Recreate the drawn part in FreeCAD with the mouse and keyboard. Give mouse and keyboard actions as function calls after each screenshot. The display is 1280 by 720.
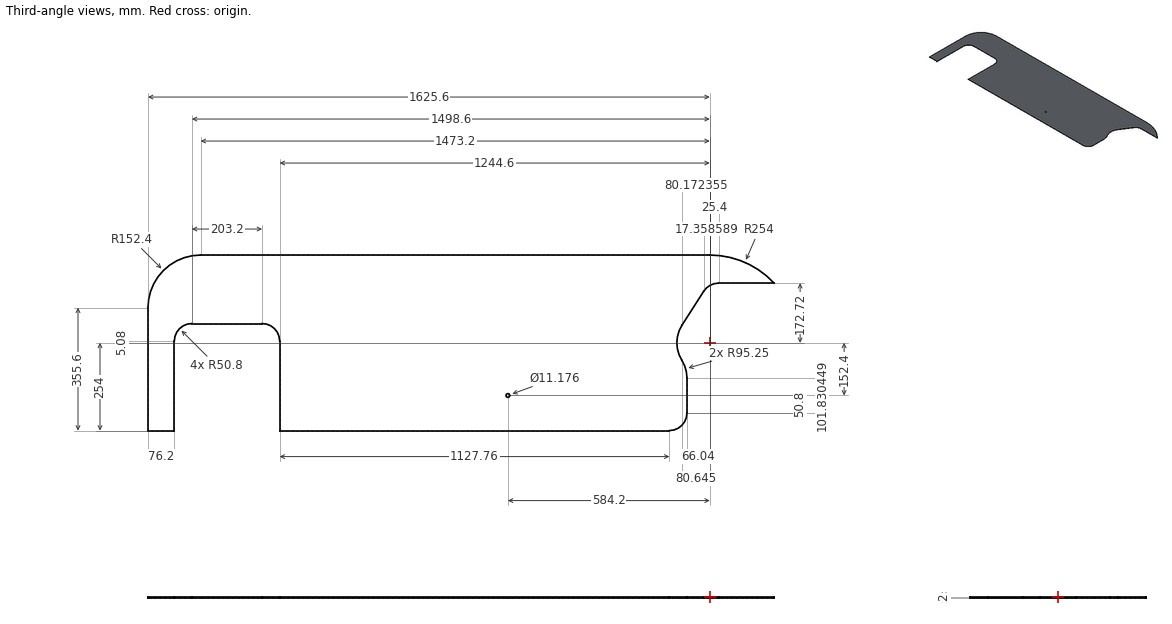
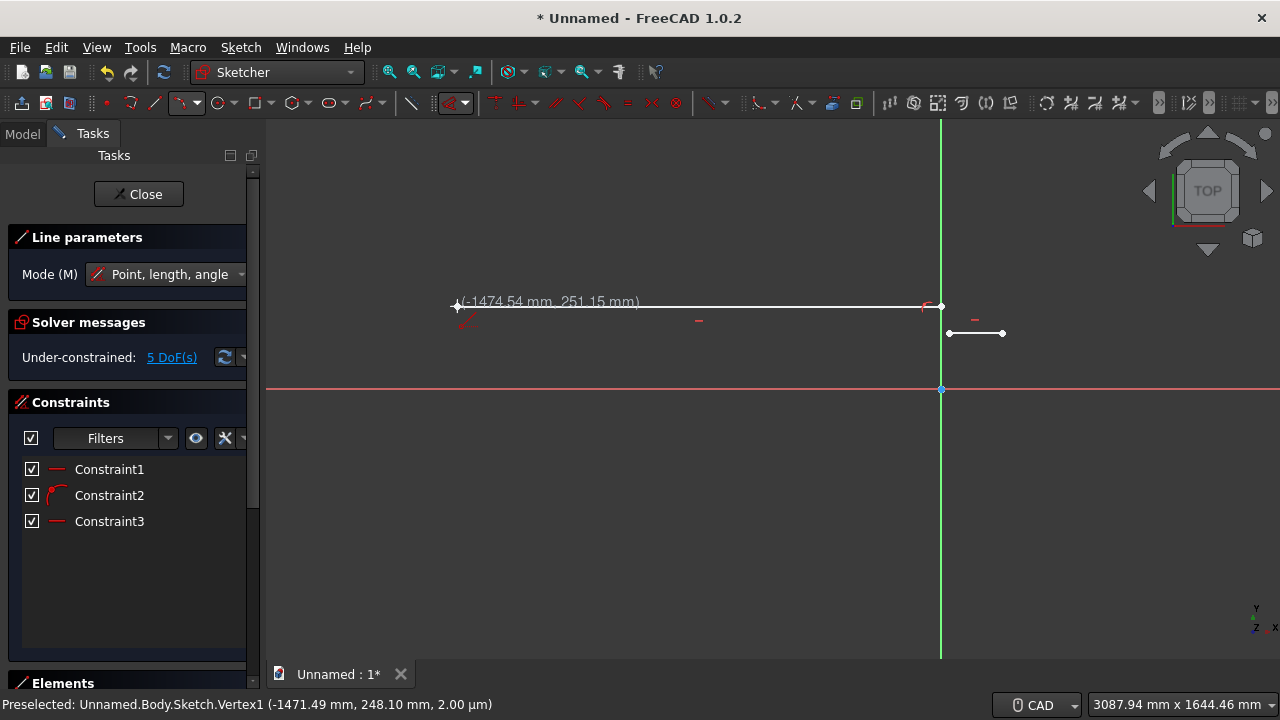
click(132, 104)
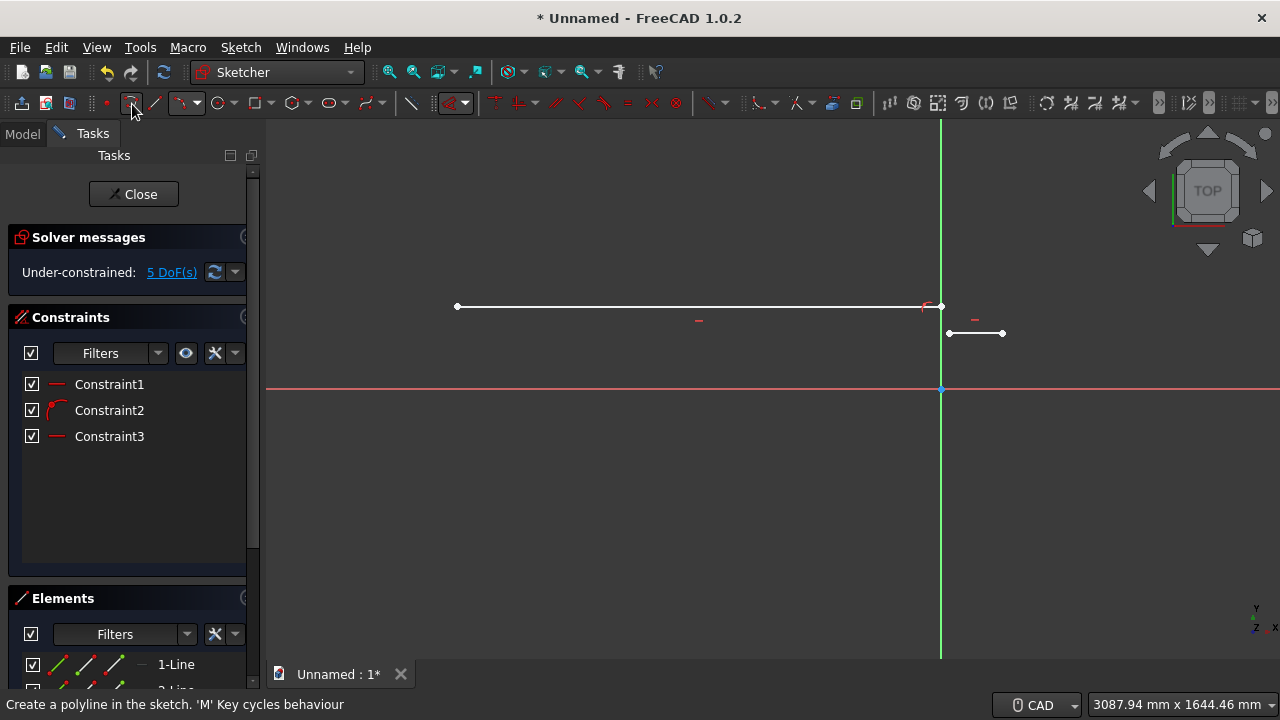
click(407, 356)
click(407, 473)
click(432, 473)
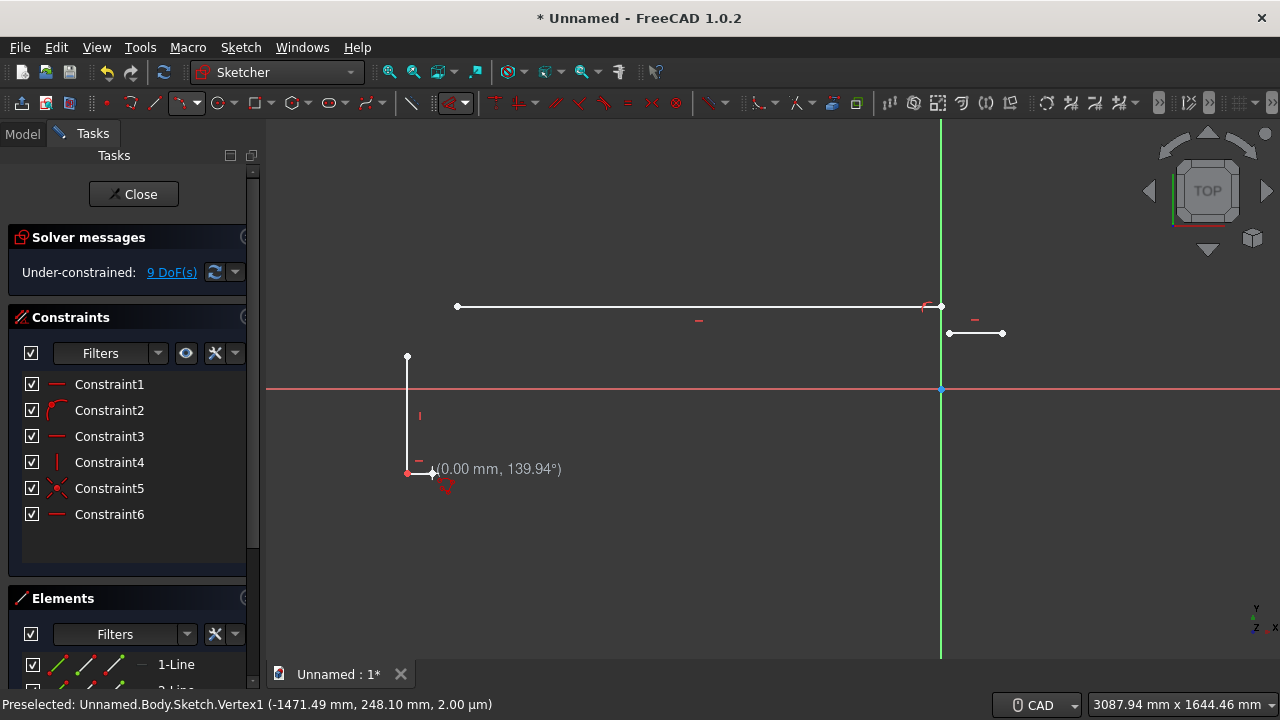
scroll(432, 388, up, 12)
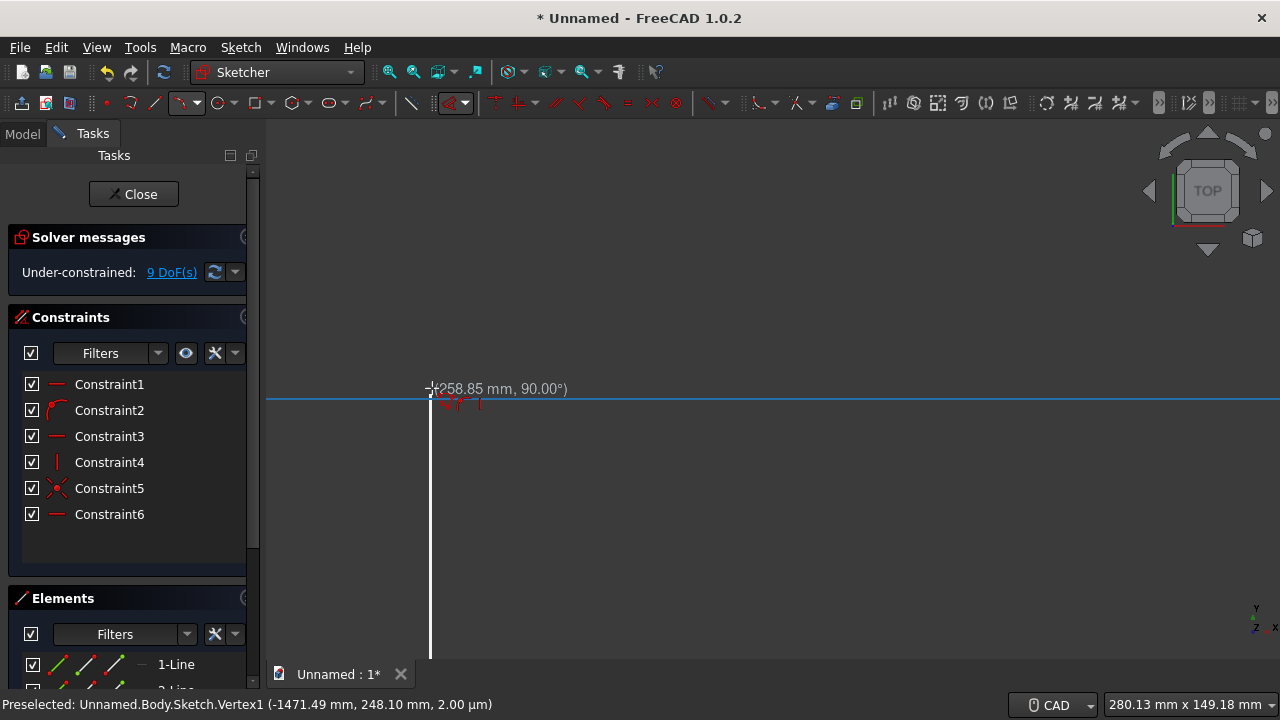
click(430, 381)
right_click(430, 381)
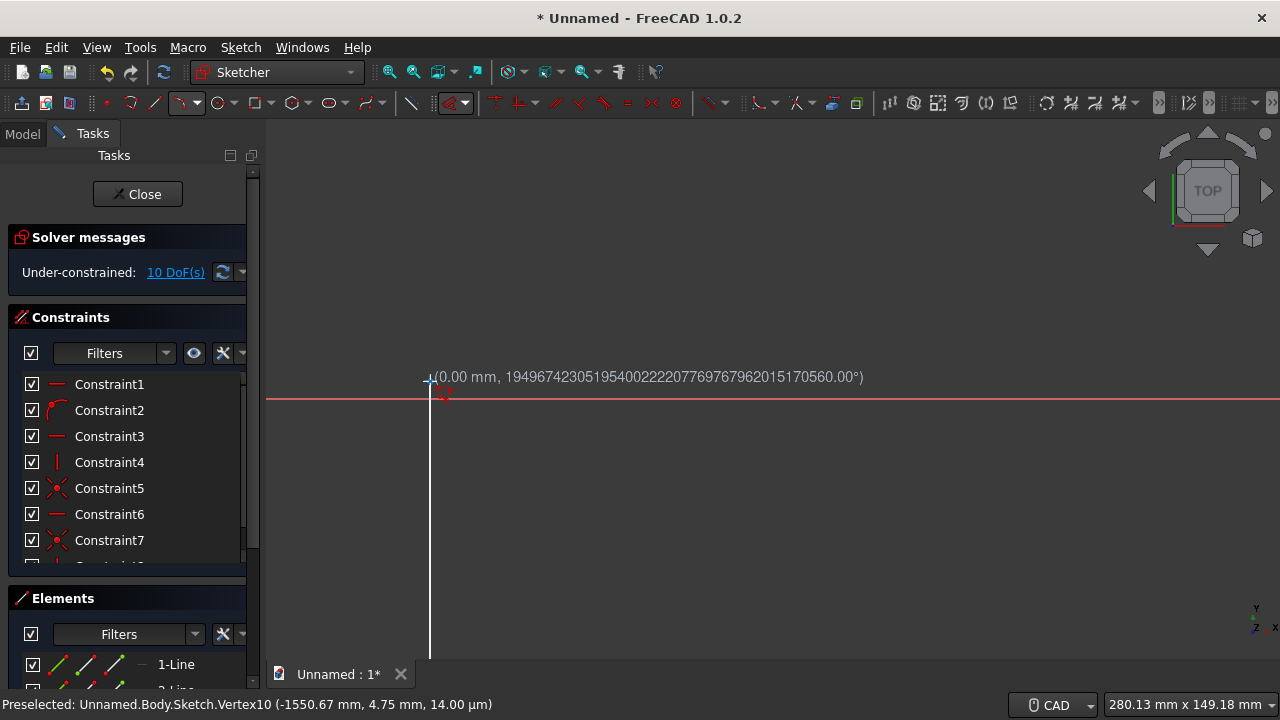
click(156, 104)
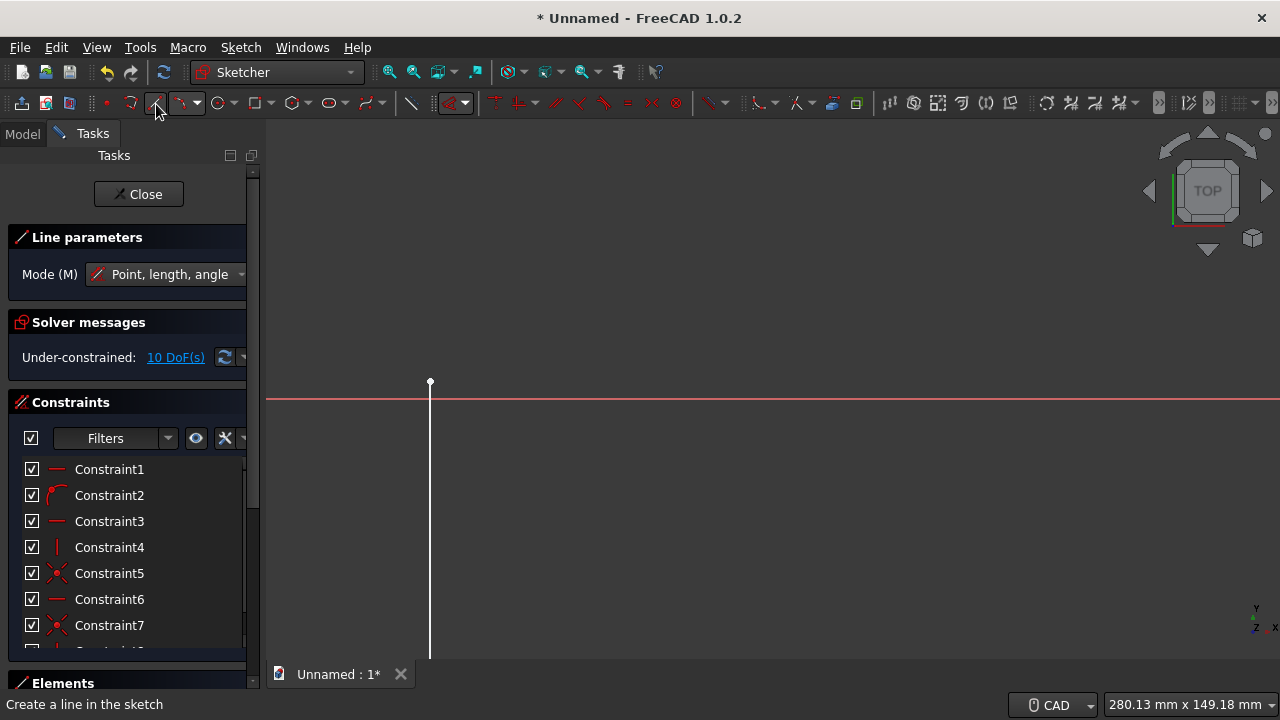
scroll(432, 388, down, 12)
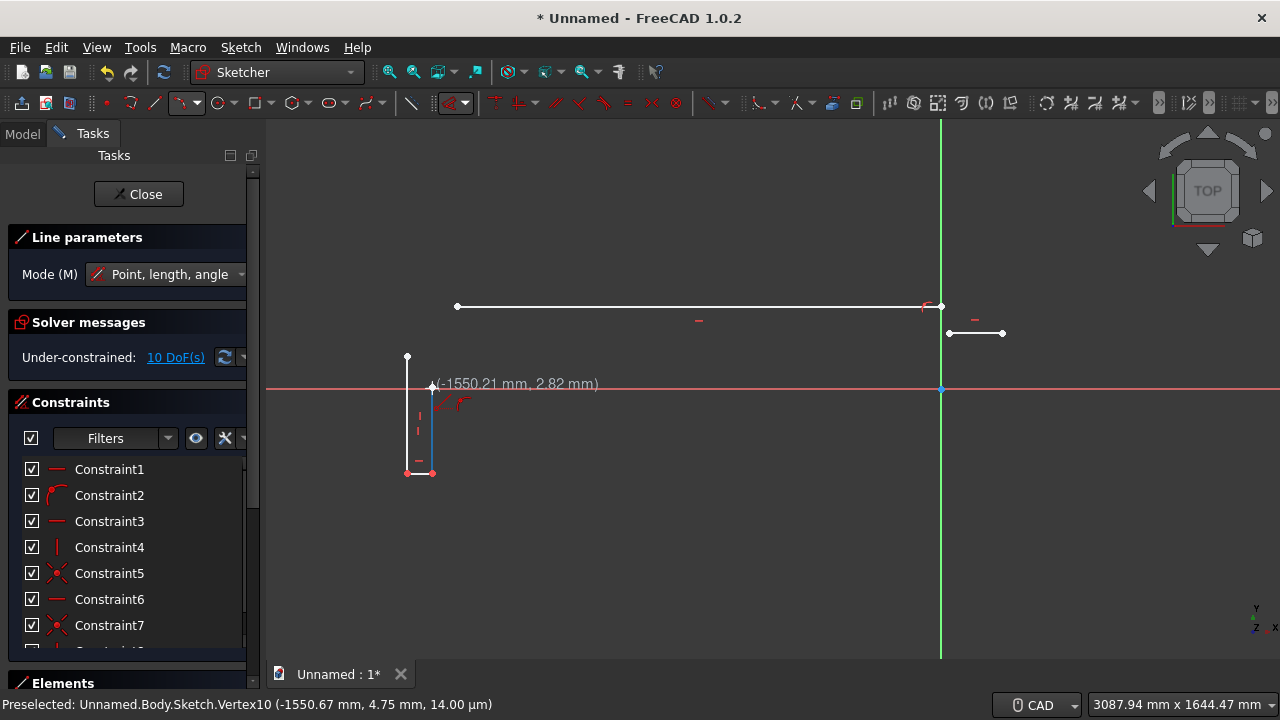
click(449, 371)
click(516, 371)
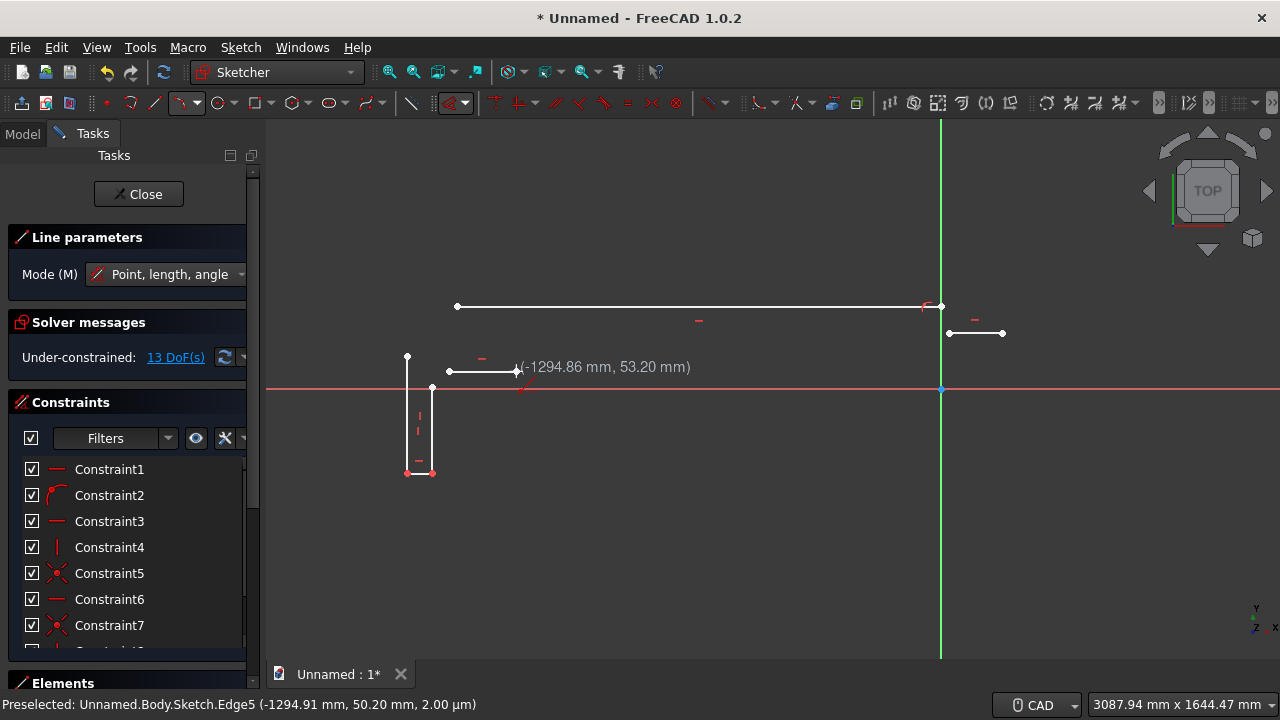
click(132, 104)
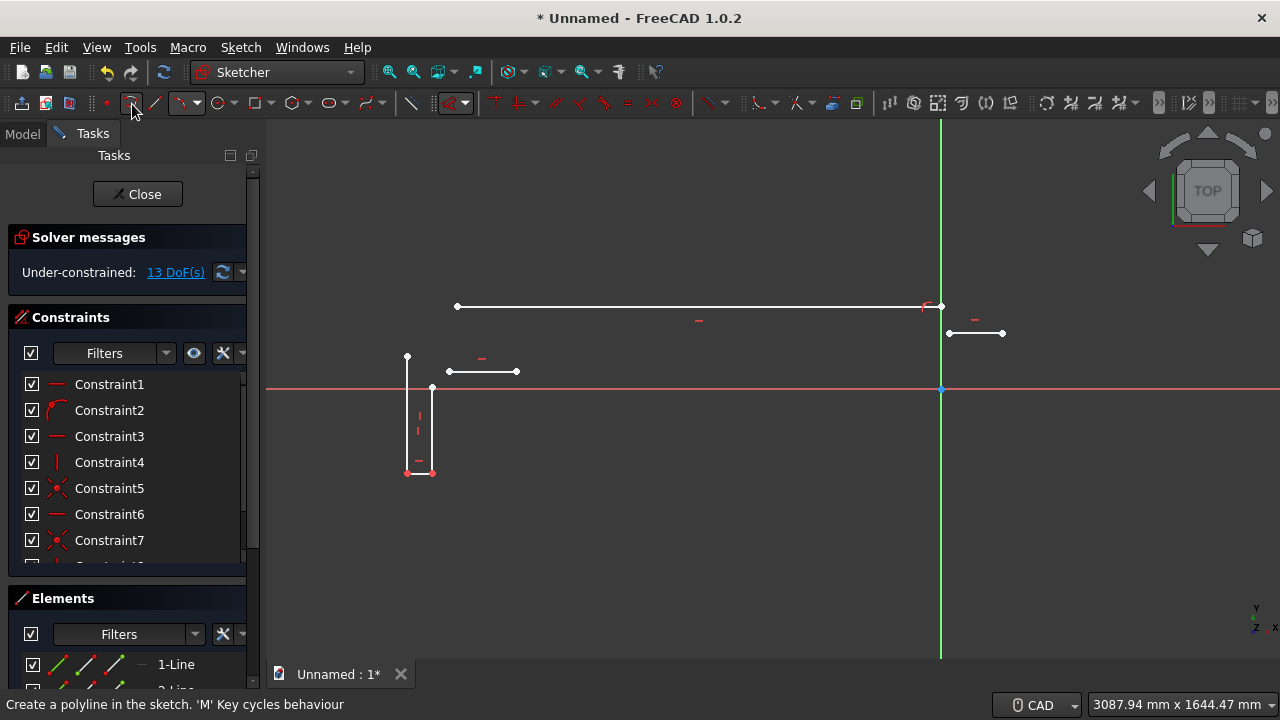
scroll(533, 388, up, 12)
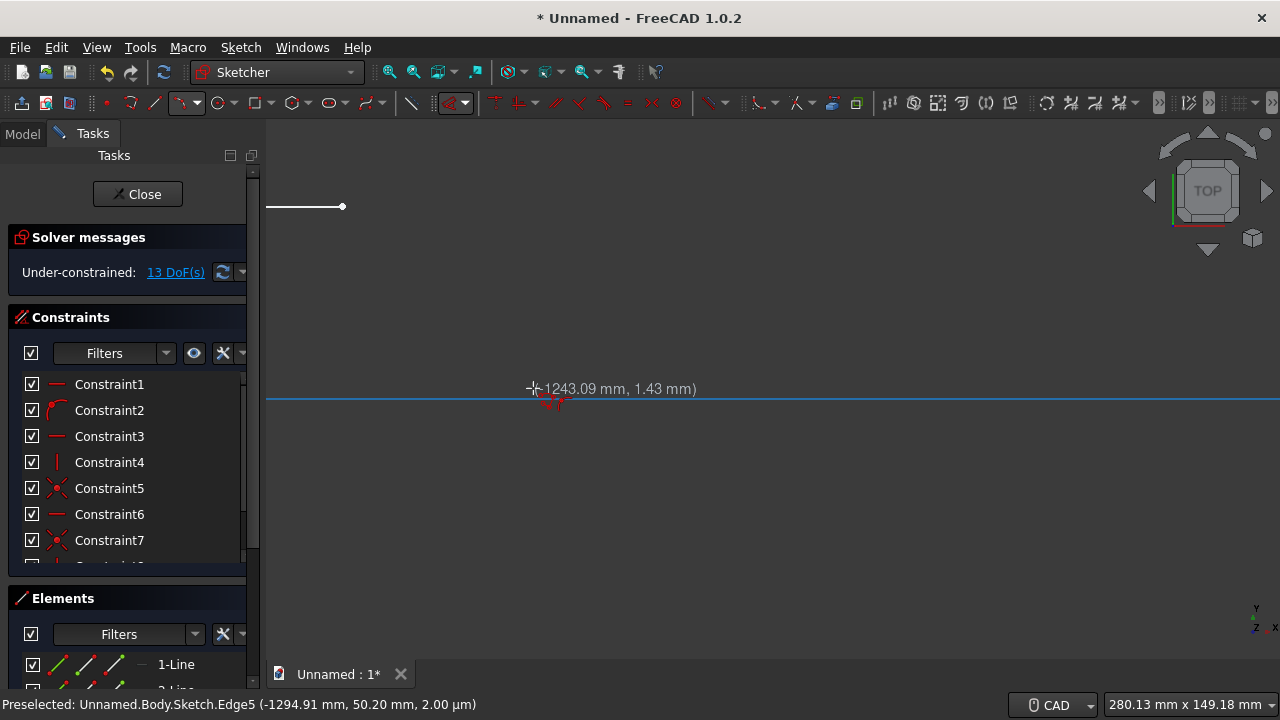
click(525, 381)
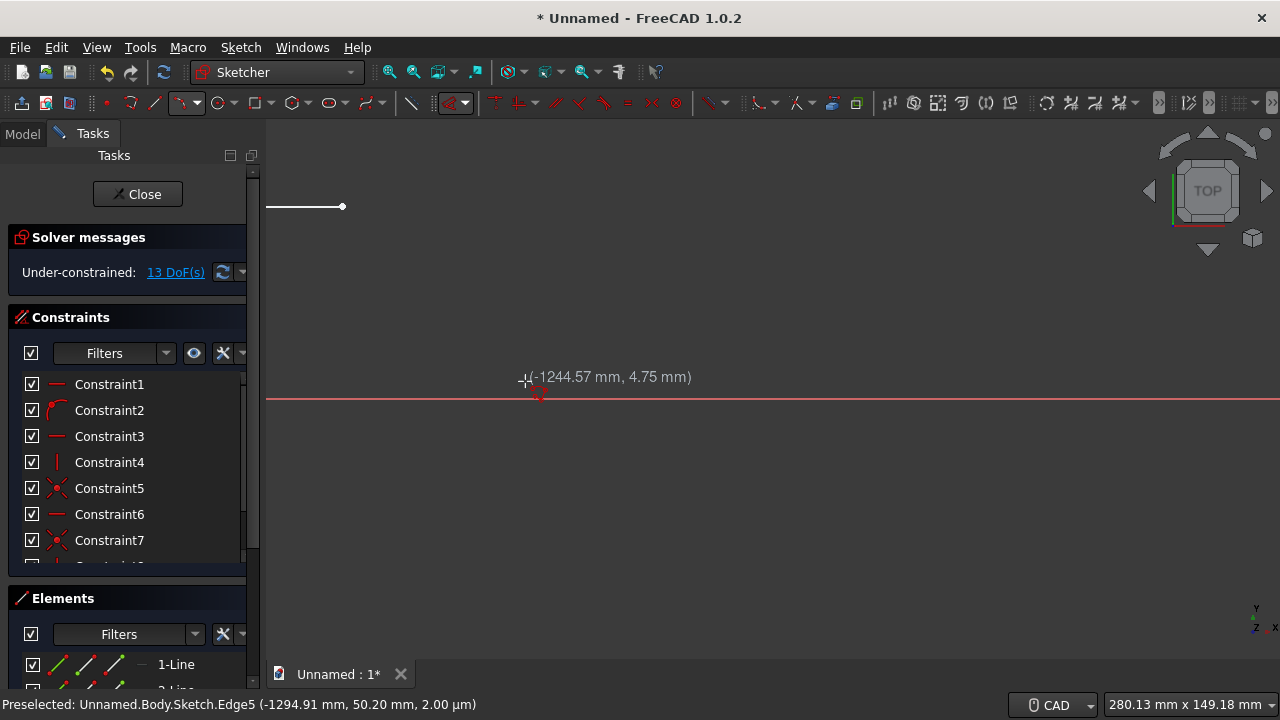
scroll(533, 388, down, 12)